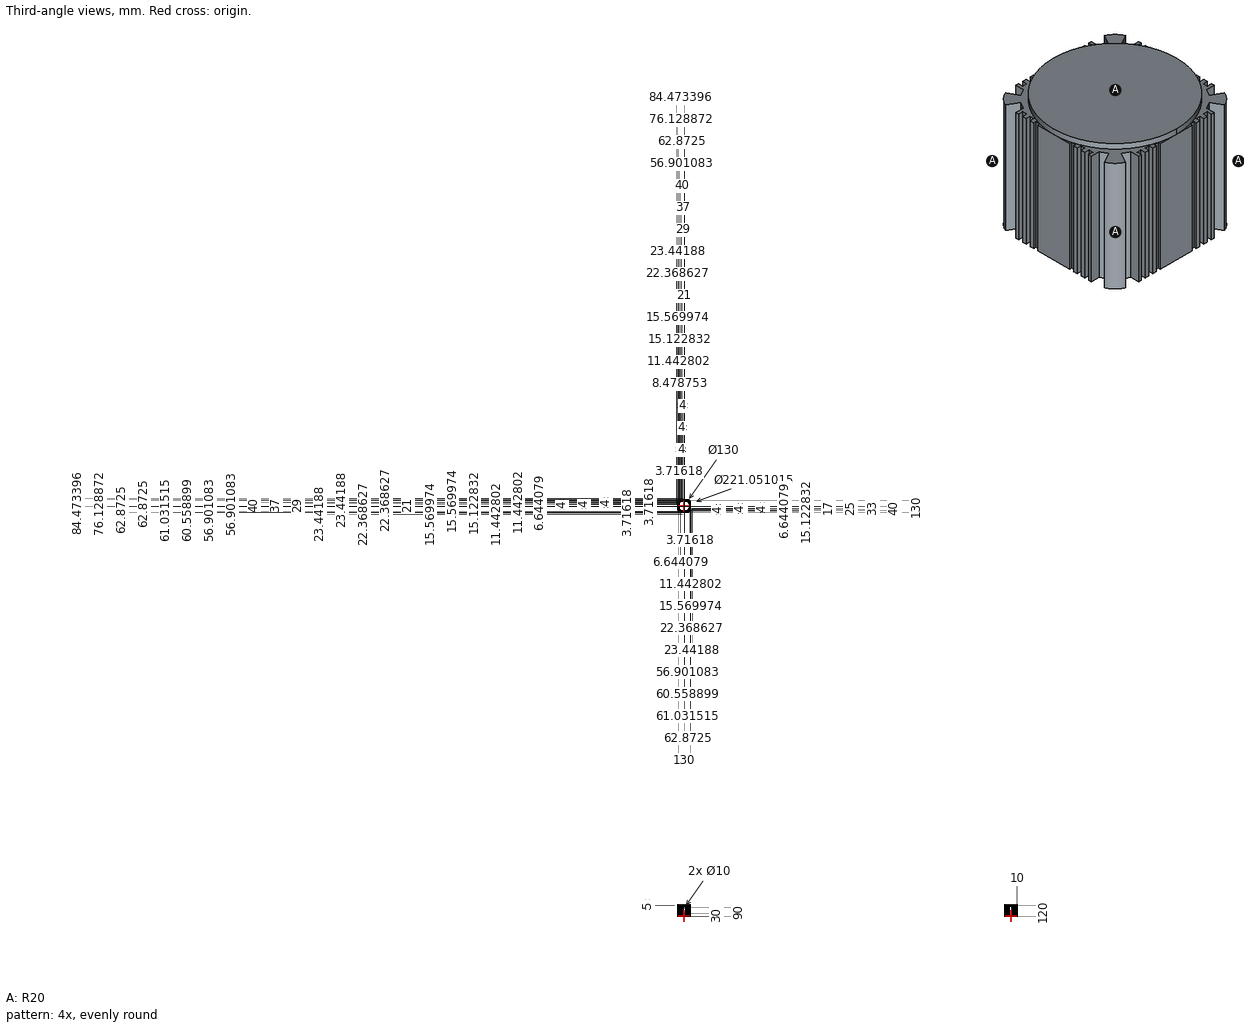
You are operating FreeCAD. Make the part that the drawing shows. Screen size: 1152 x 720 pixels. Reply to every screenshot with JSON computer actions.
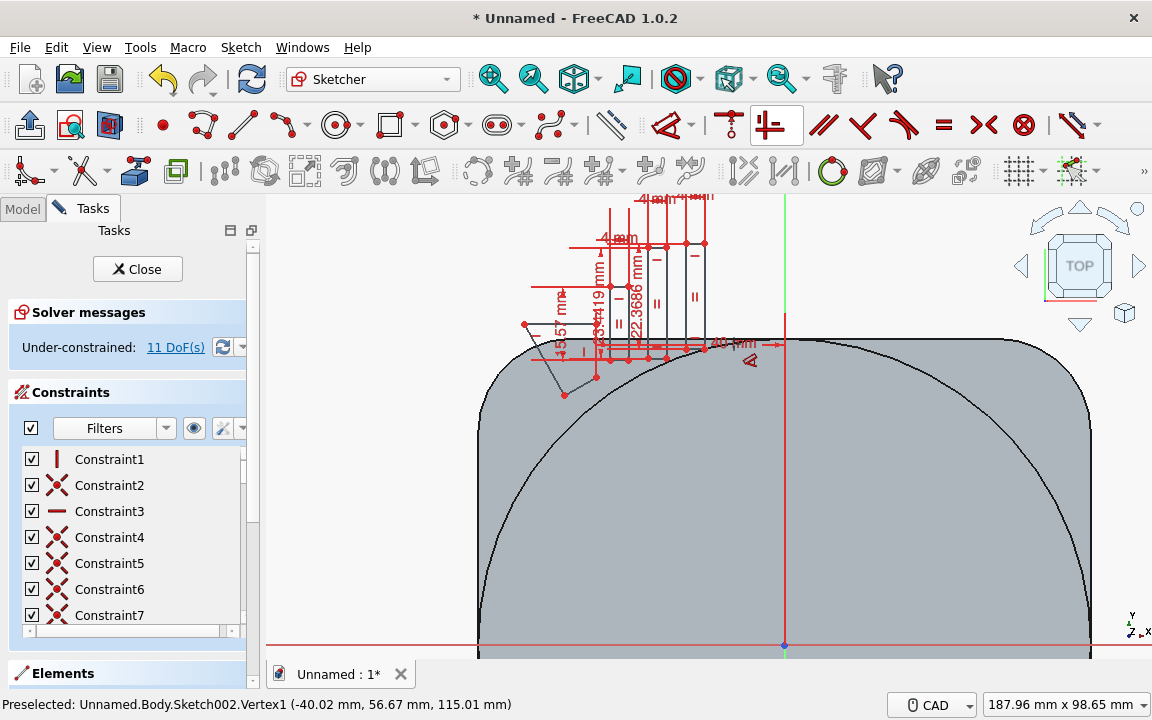
{"action": "left_click", "coordinate": [610, 287]}
{"action": "left_click", "coordinate": [737, 253]}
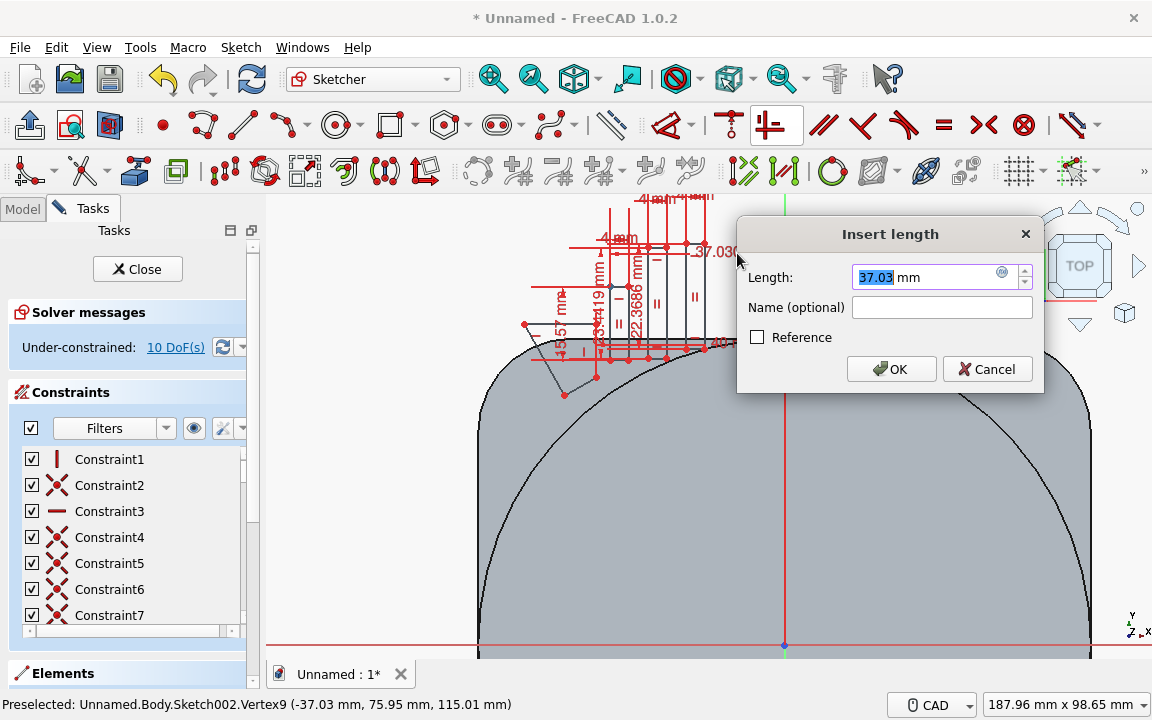
{"action": "type", "text": "37"}
{"action": "key", "text": "Return"}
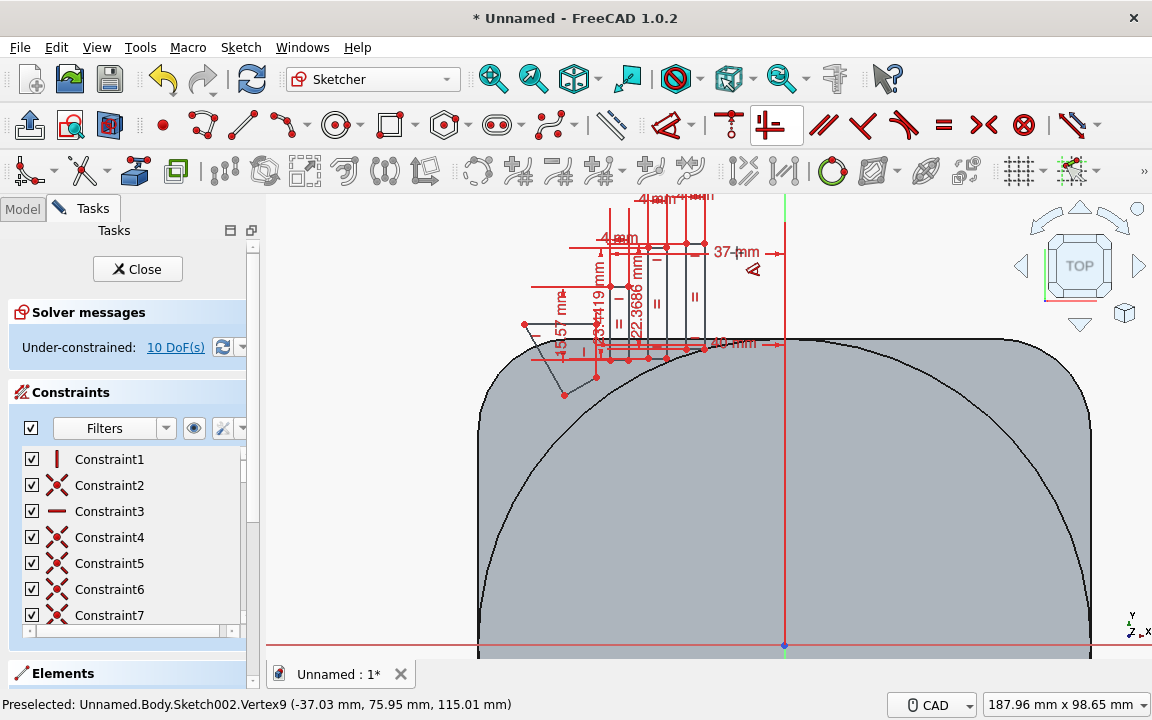
{"action": "left_click", "coordinate": [648, 248]}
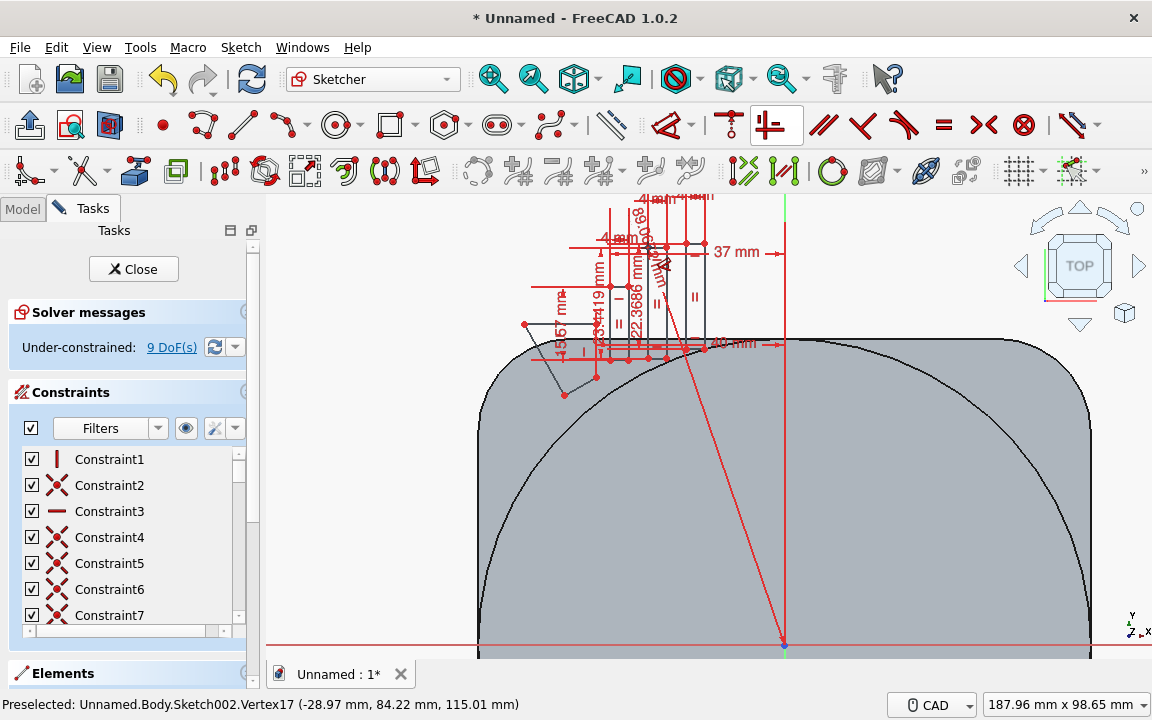
{"action": "key", "text": "Escape"}
{"action": "key", "text": "Escape"}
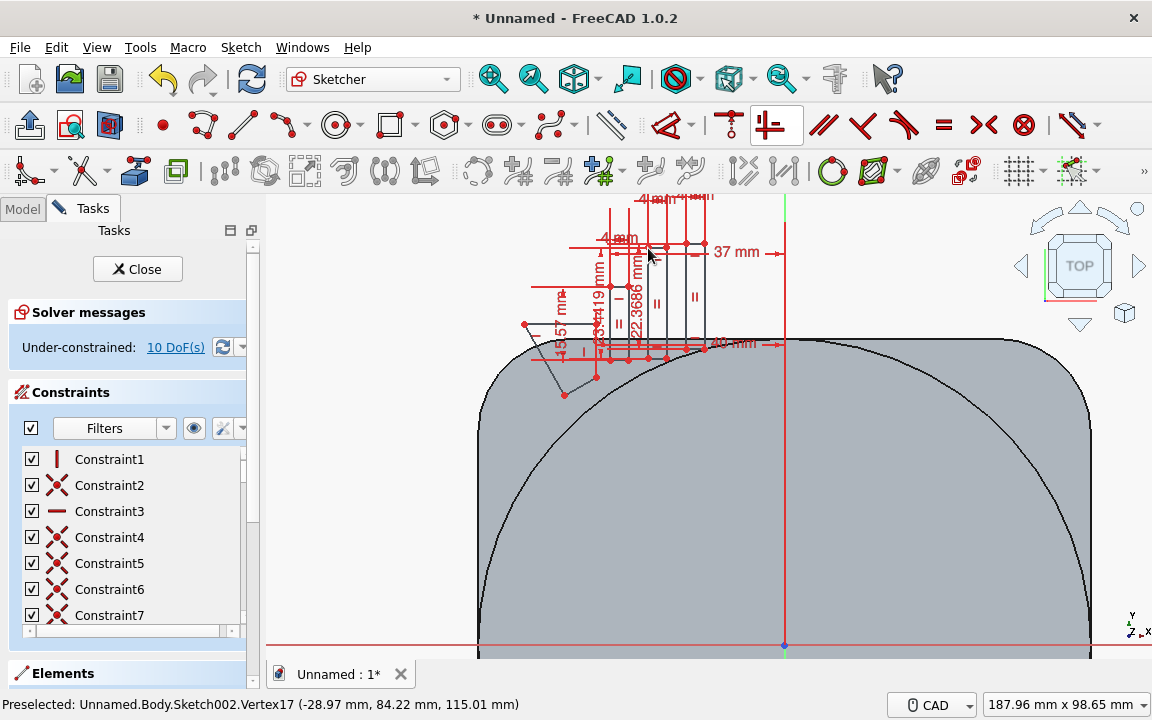
{"action": "left_click", "coordinate": [648, 248]}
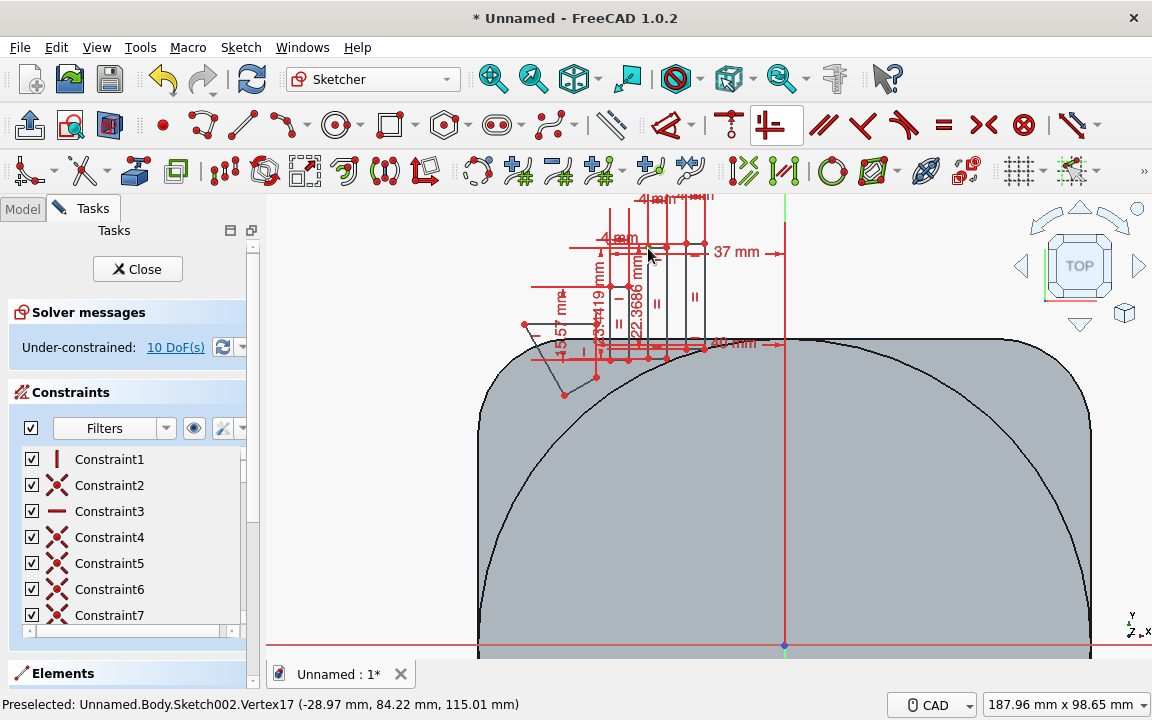
{"action": "left_click", "coordinate": [694, 126]}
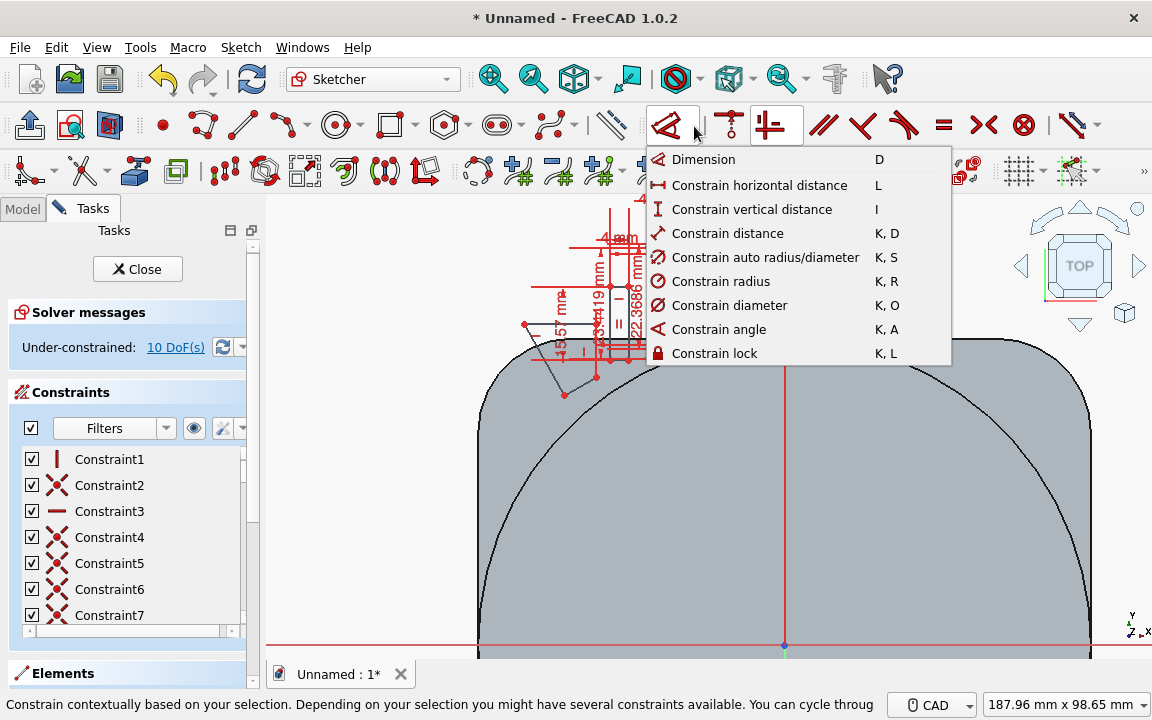
{"action": "left_click", "coordinate": [799, 185]}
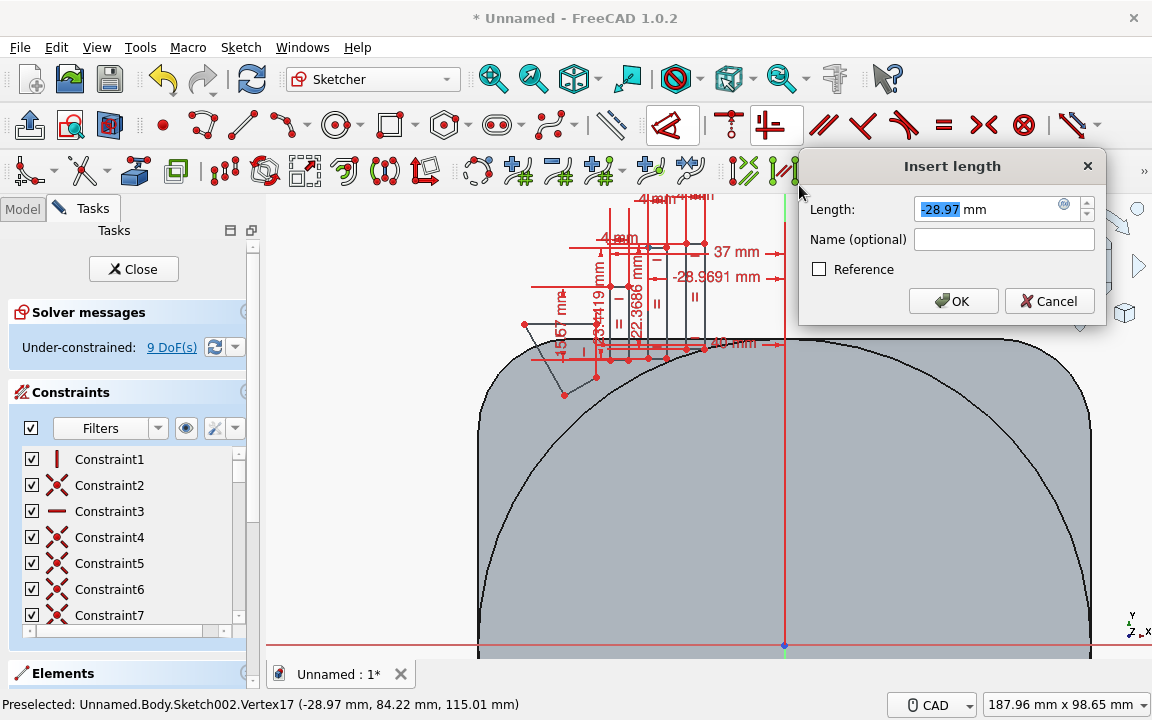
{"action": "type", "text": "-29"}
{"action": "key", "text": "Return"}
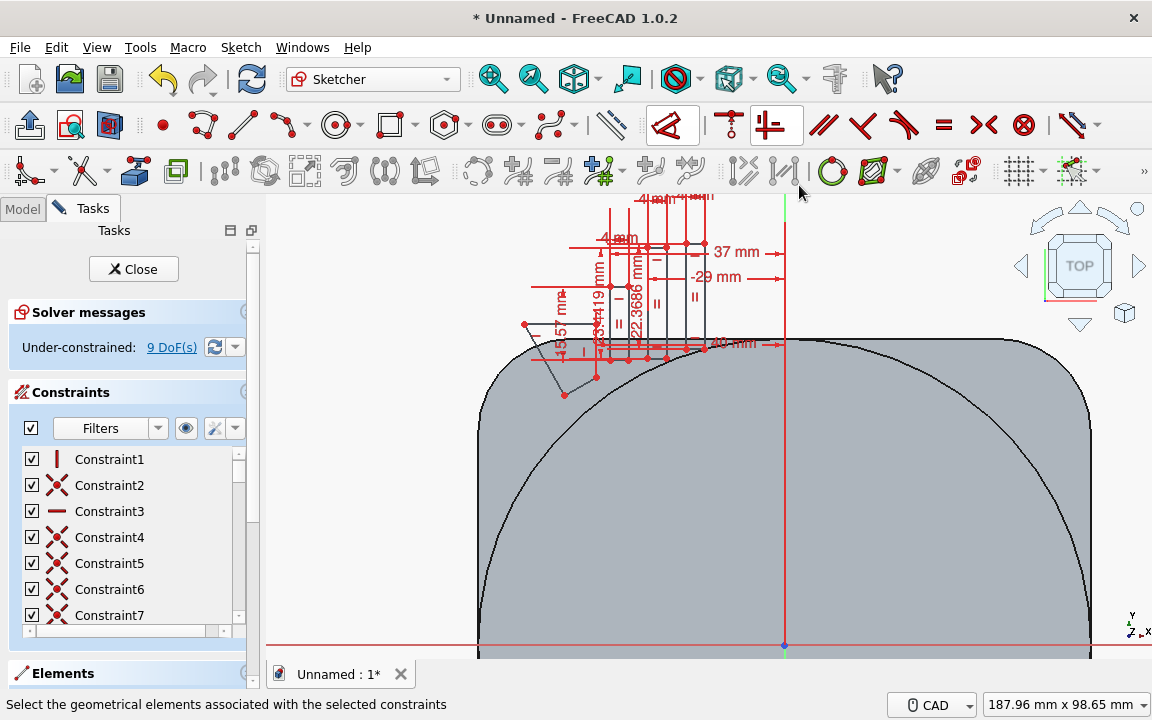
{"action": "left_click", "coordinate": [686, 244]}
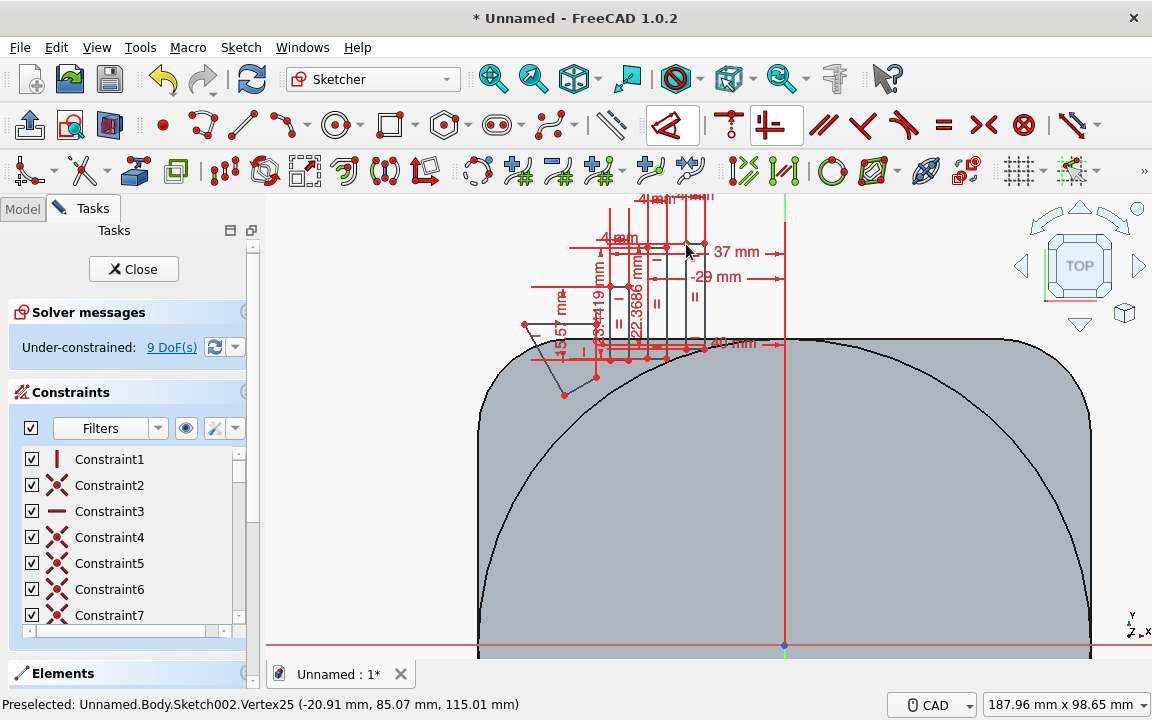
{"action": "key", "text": "l"}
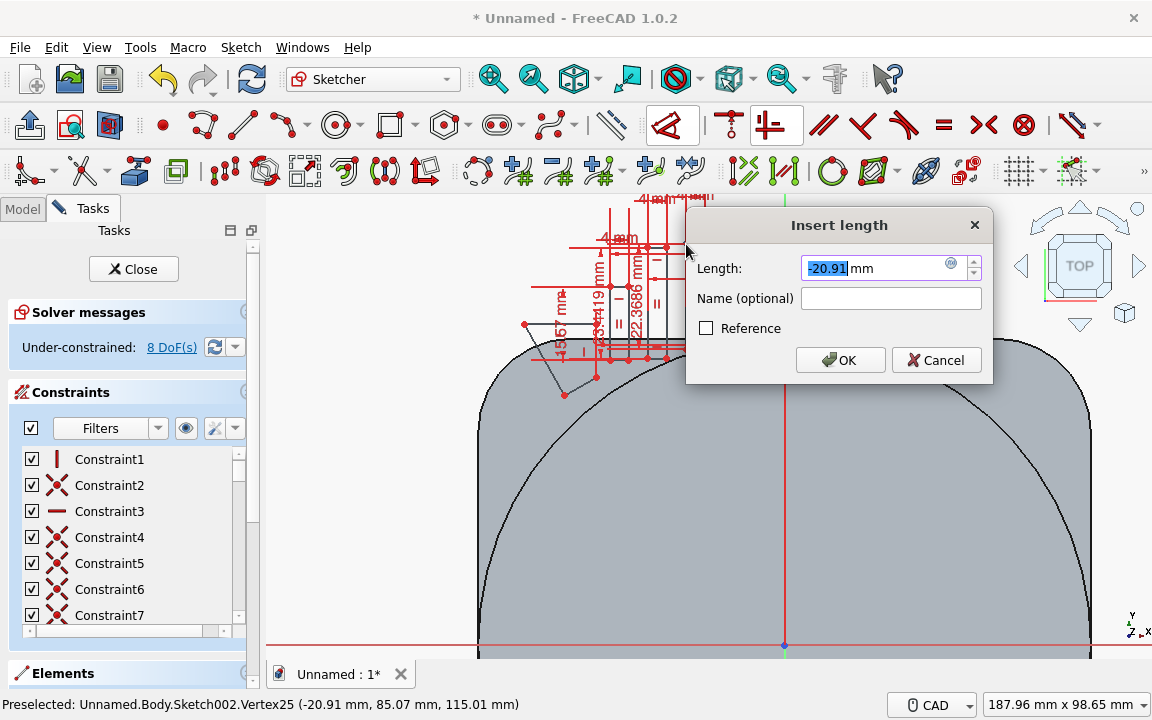
{"action": "type", "text": "-21"}
{"action": "key", "text": "Return"}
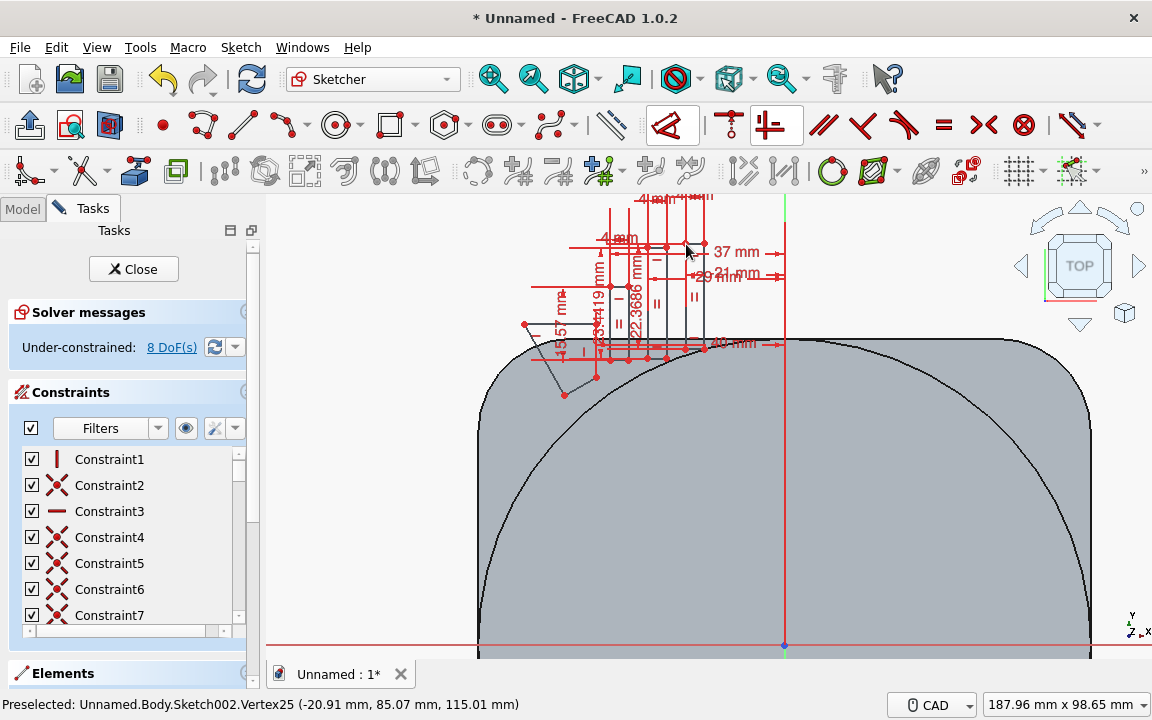
{"action": "left_click", "coordinate": [686, 349]}